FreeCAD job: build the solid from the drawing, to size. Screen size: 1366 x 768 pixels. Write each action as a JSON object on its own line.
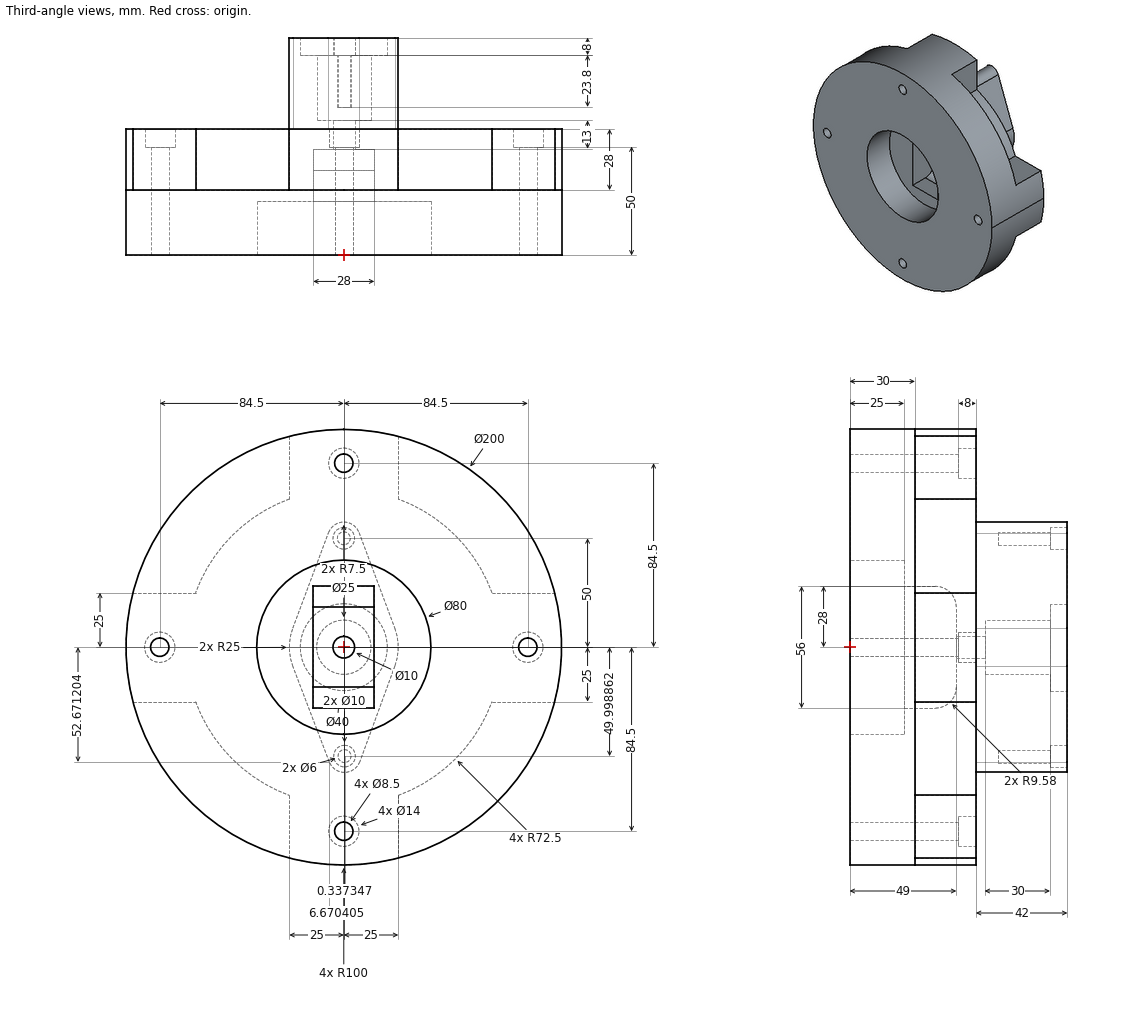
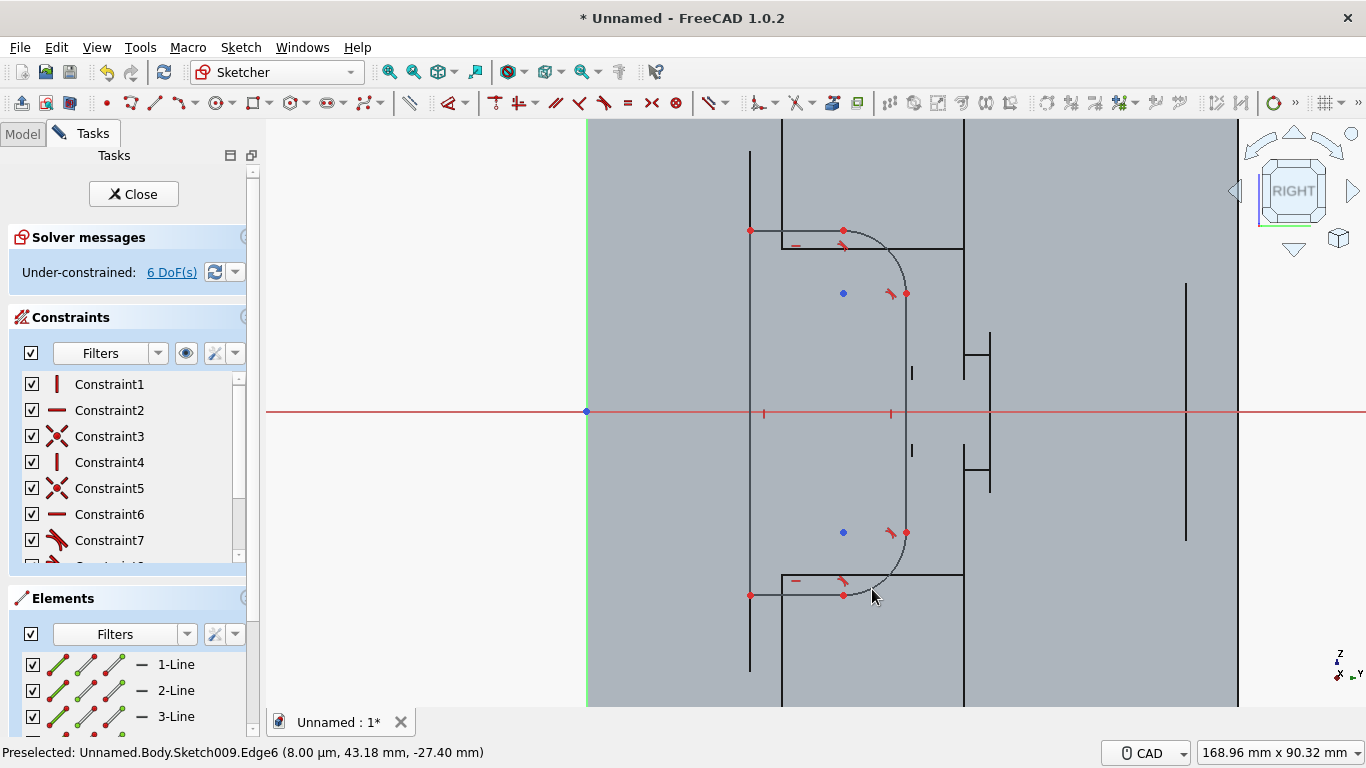
{"action": "left_click", "coordinate": [899, 265]}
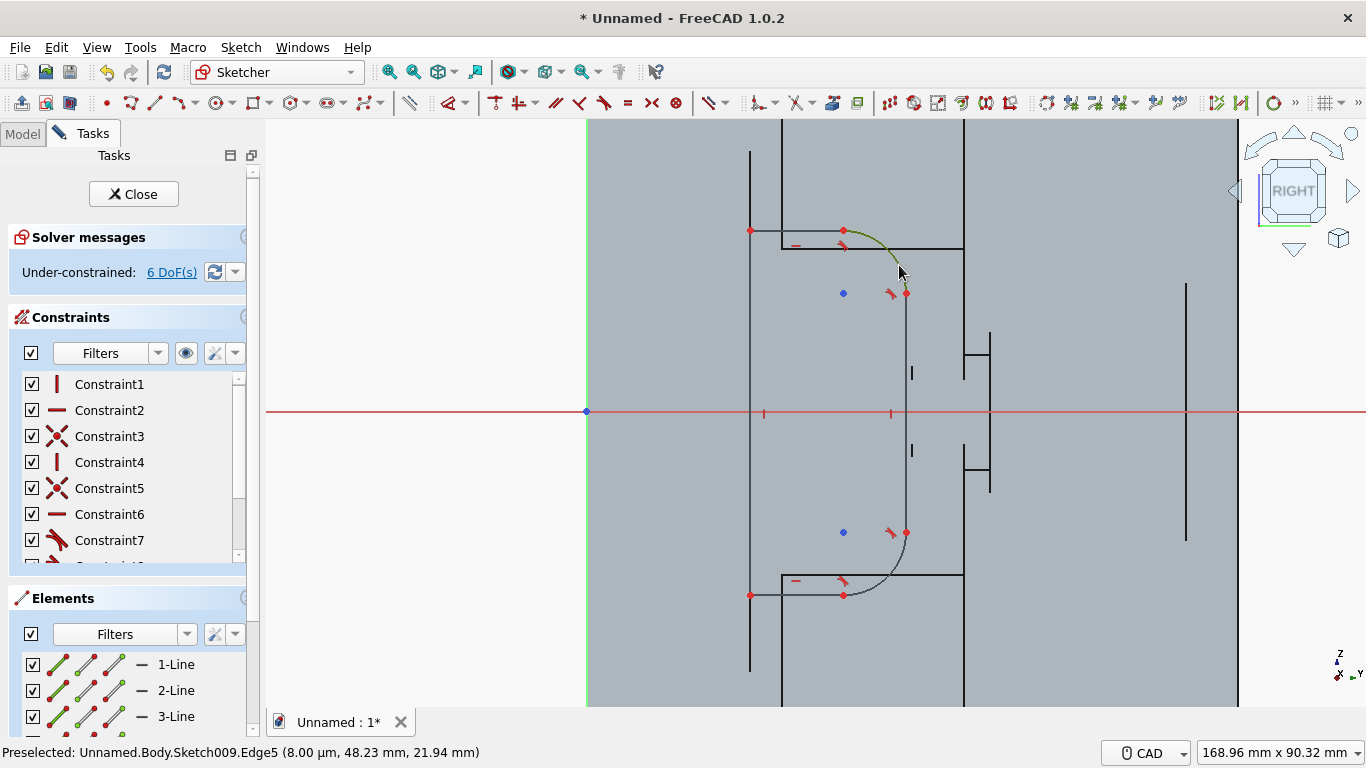
{"action": "left_click", "coordinate": [872, 589]}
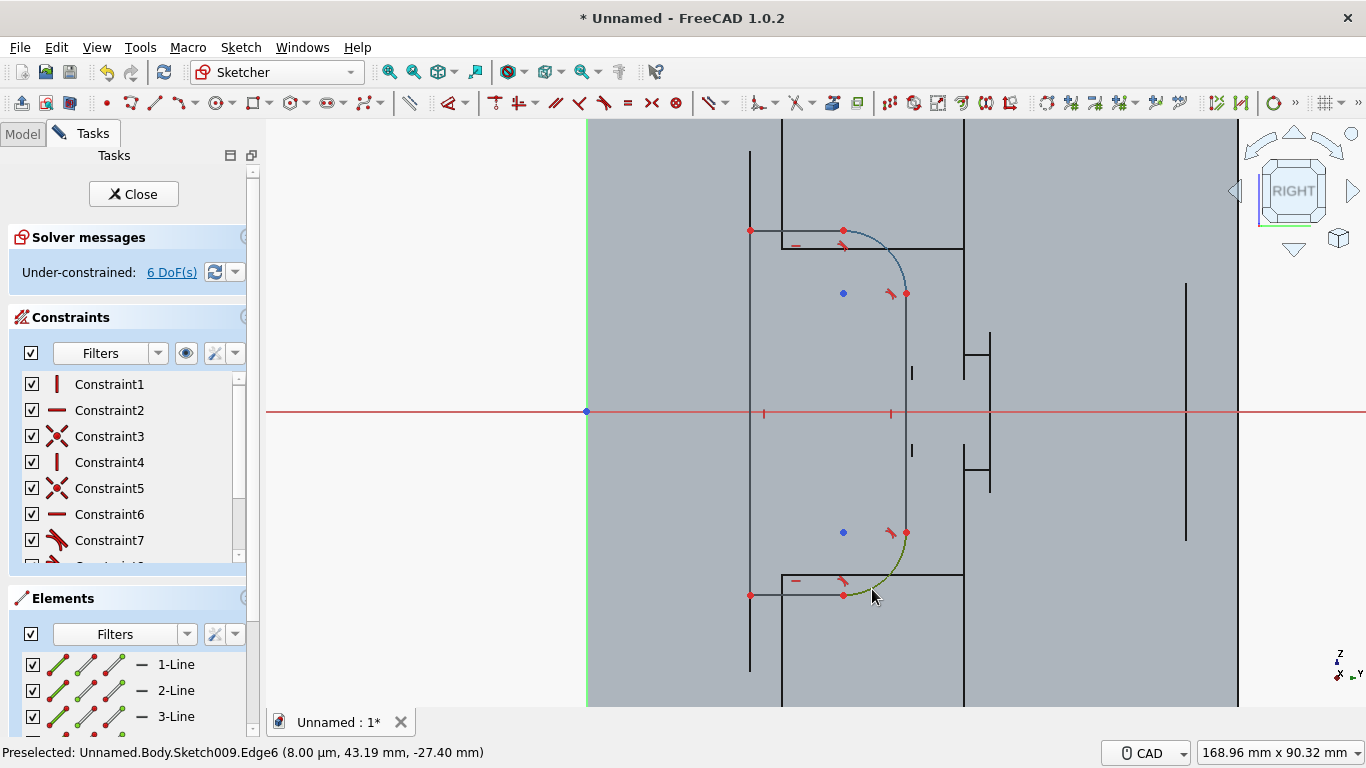
{"action": "key", "text": "e"}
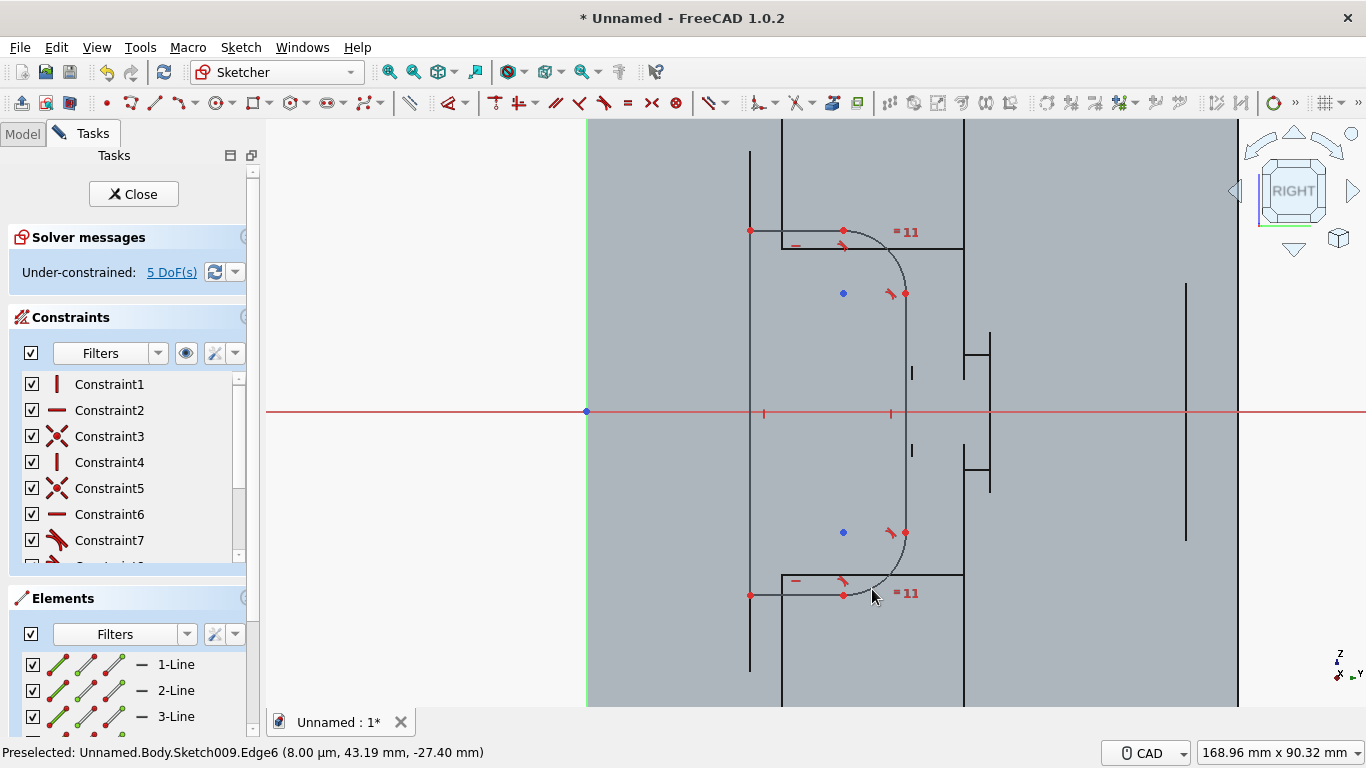
{"action": "left_click", "coordinate": [448, 104]}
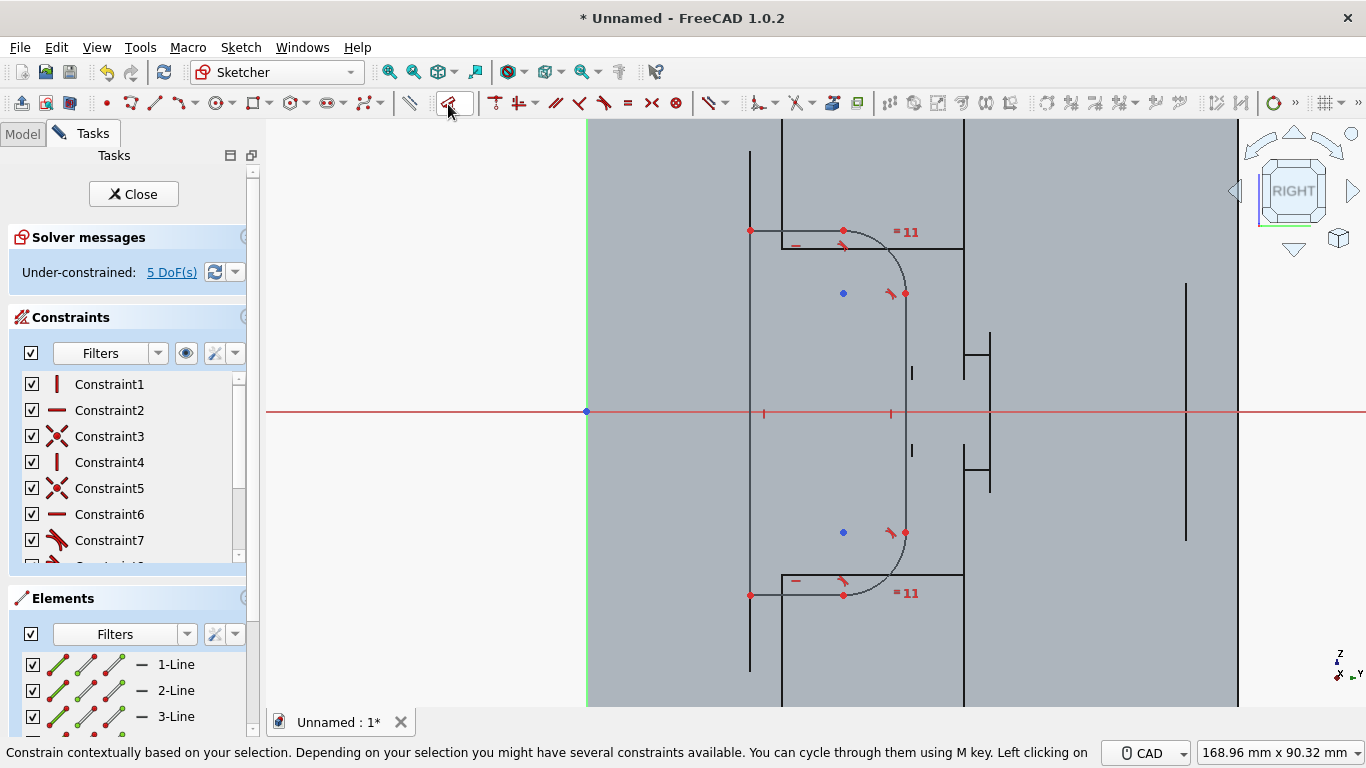
{"action": "left_click", "coordinate": [899, 265]}
{"action": "left_click", "coordinate": [927, 250]}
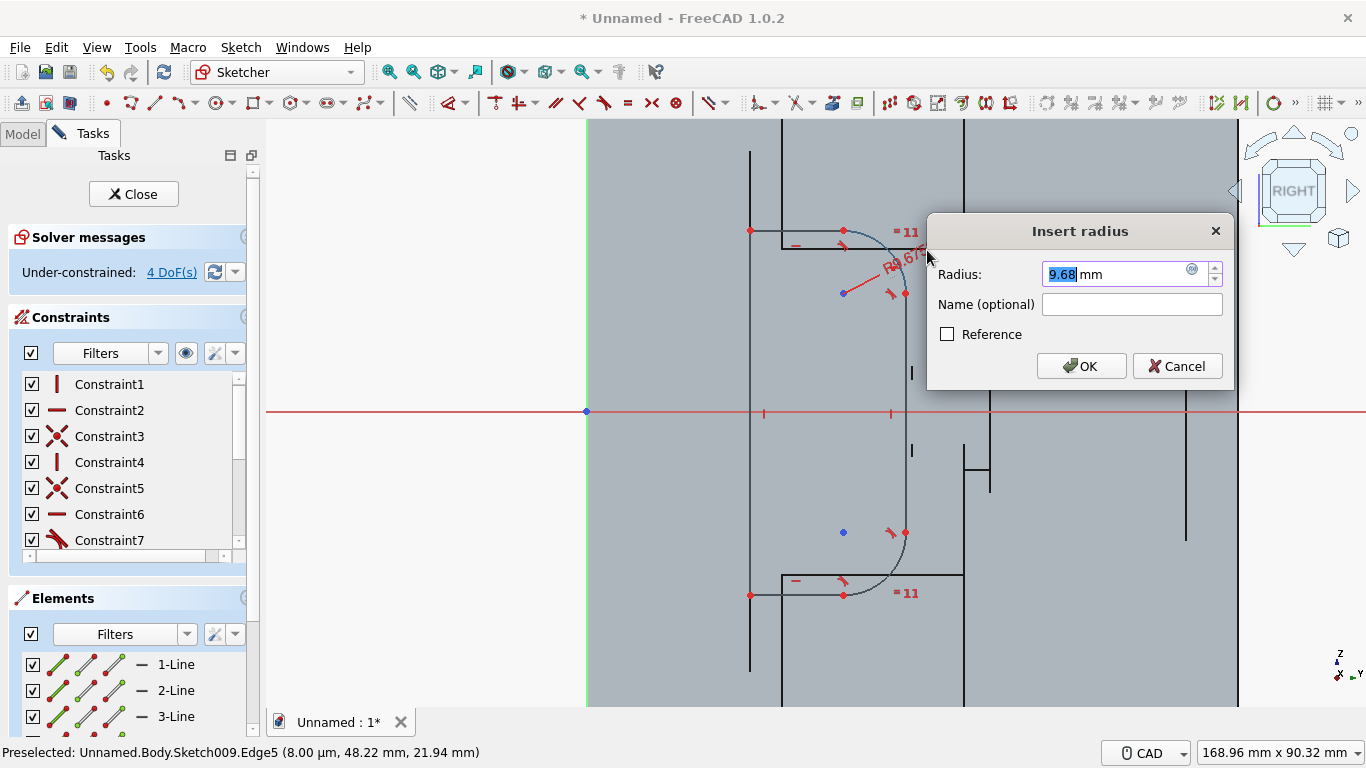
{"action": "type", "text": "9.58"}
{"action": "key", "text": "Return"}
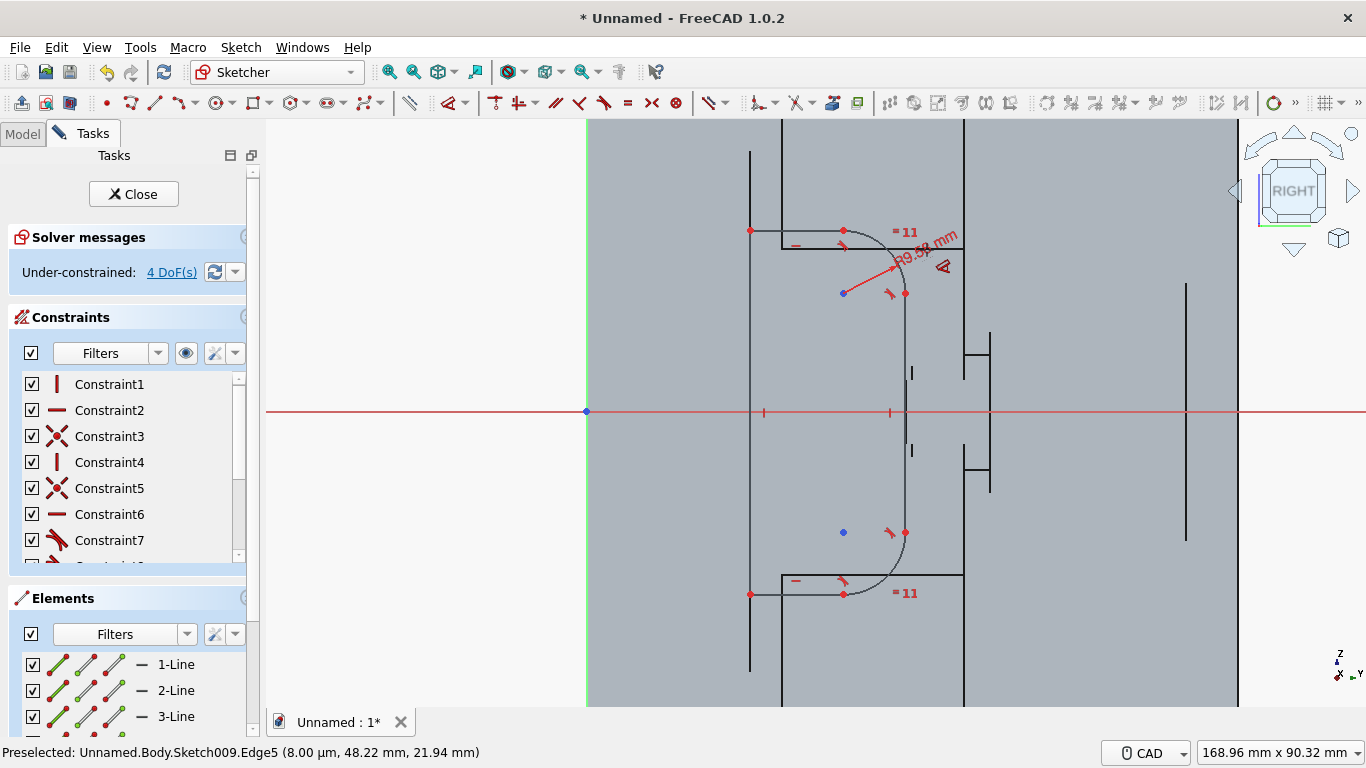
{"action": "left_click", "coordinate": [750, 340]}
{"action": "left_click", "coordinate": [784, 329]}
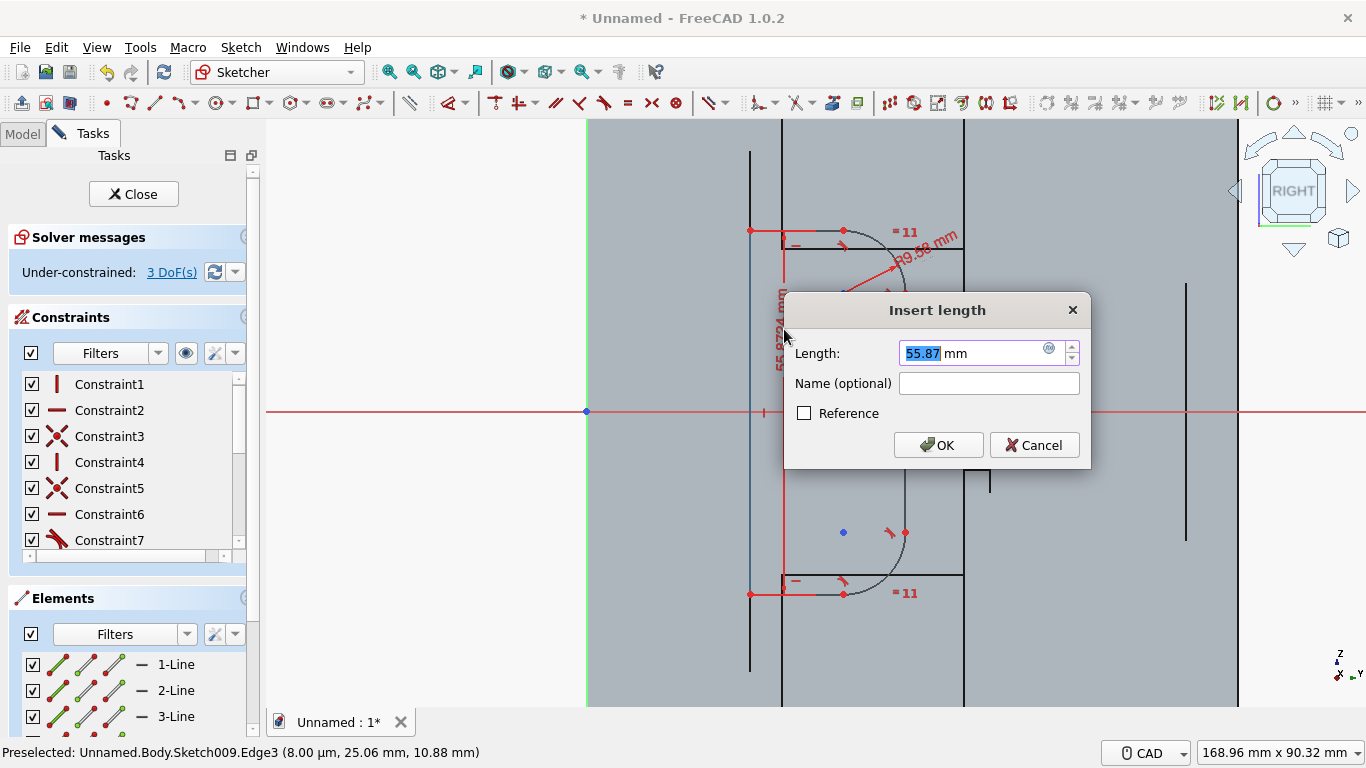
{"action": "type", "text": "56"}
{"action": "key", "text": "Return"}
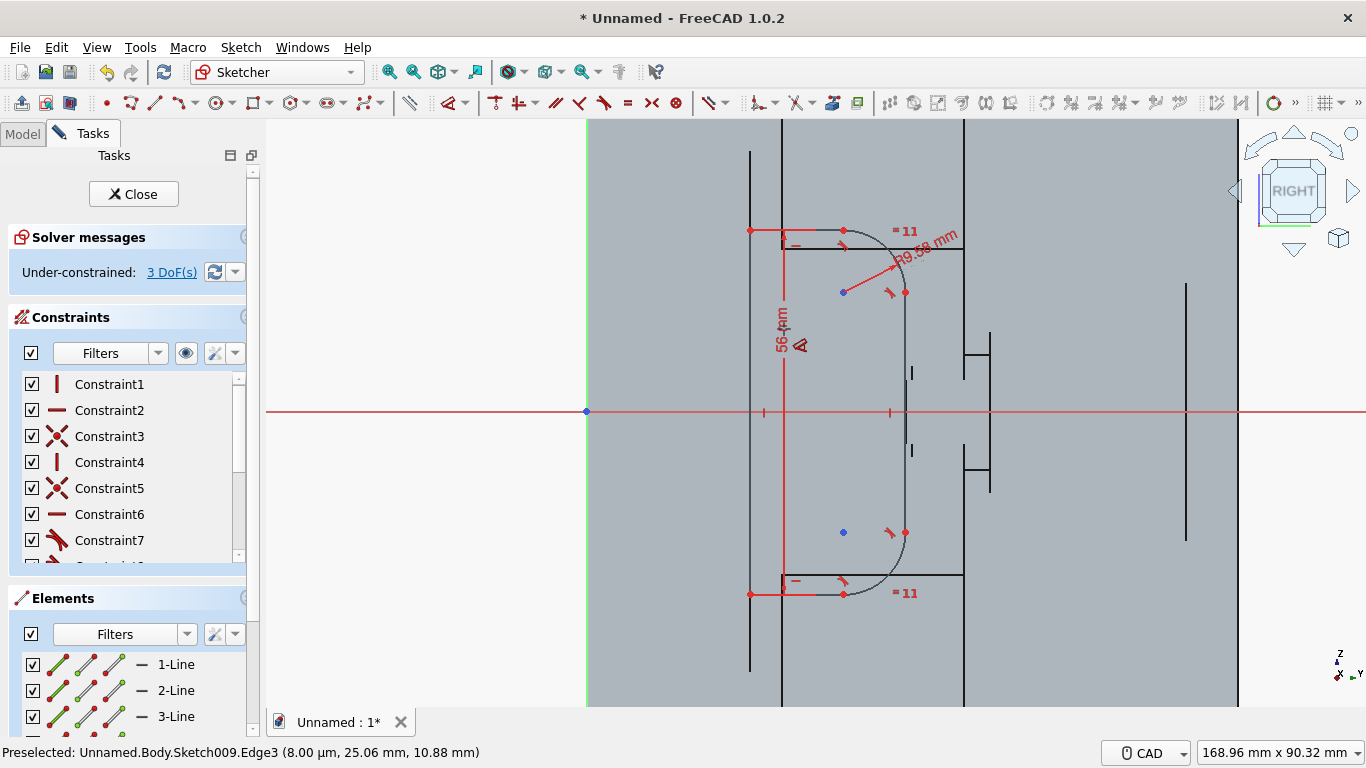
{"action": "left_click", "coordinate": [905, 533]}
{"action": "left_click", "coordinate": [673, 567]}